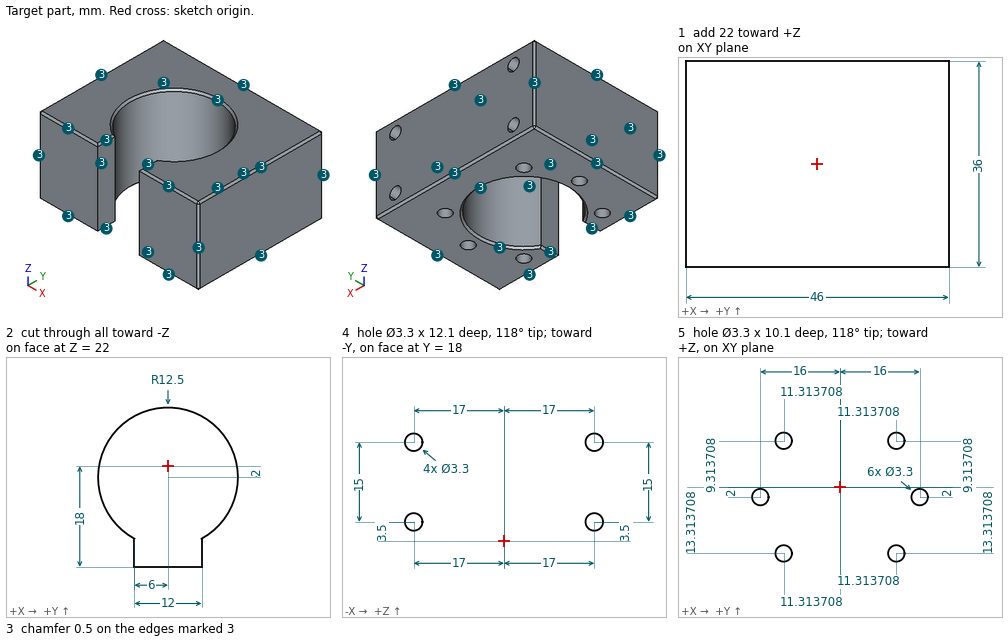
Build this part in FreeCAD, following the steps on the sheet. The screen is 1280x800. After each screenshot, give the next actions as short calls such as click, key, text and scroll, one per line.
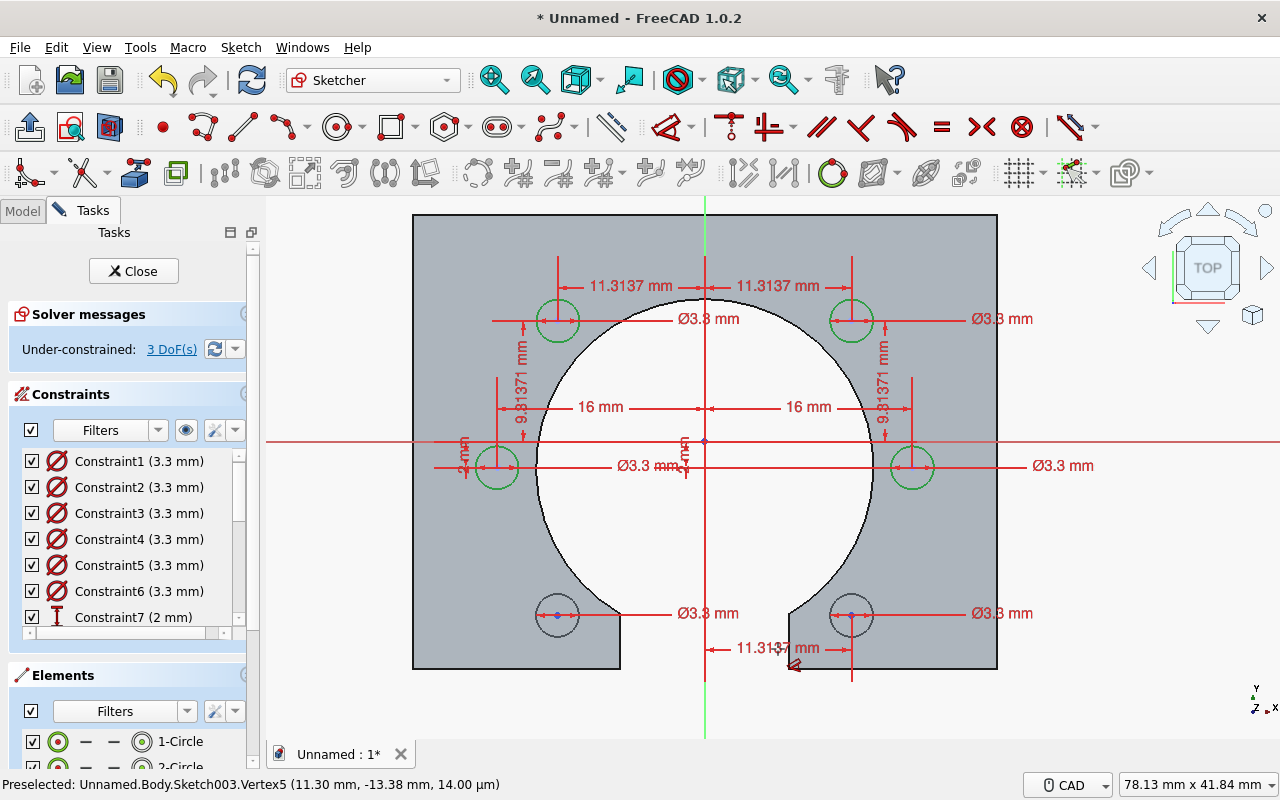
click(852, 615)
click(886, 529)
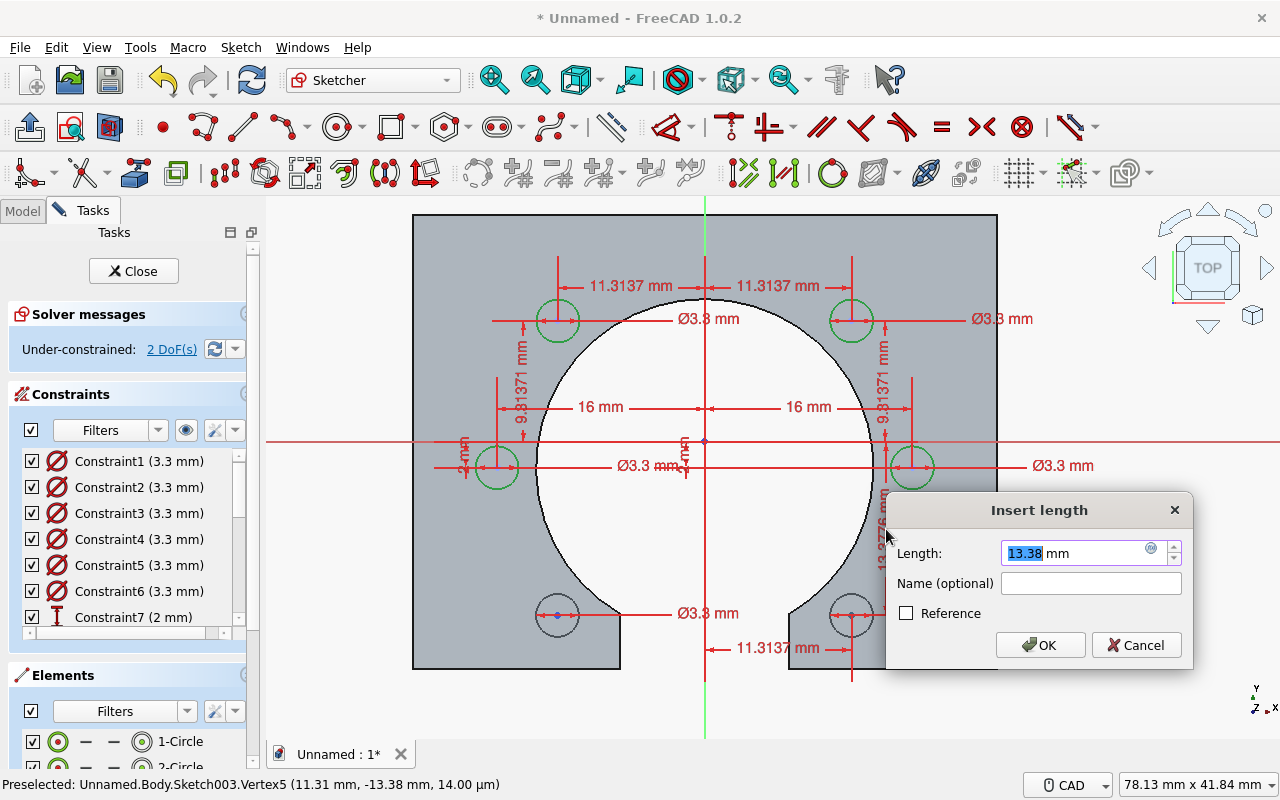
text(13.313708)
key(Return)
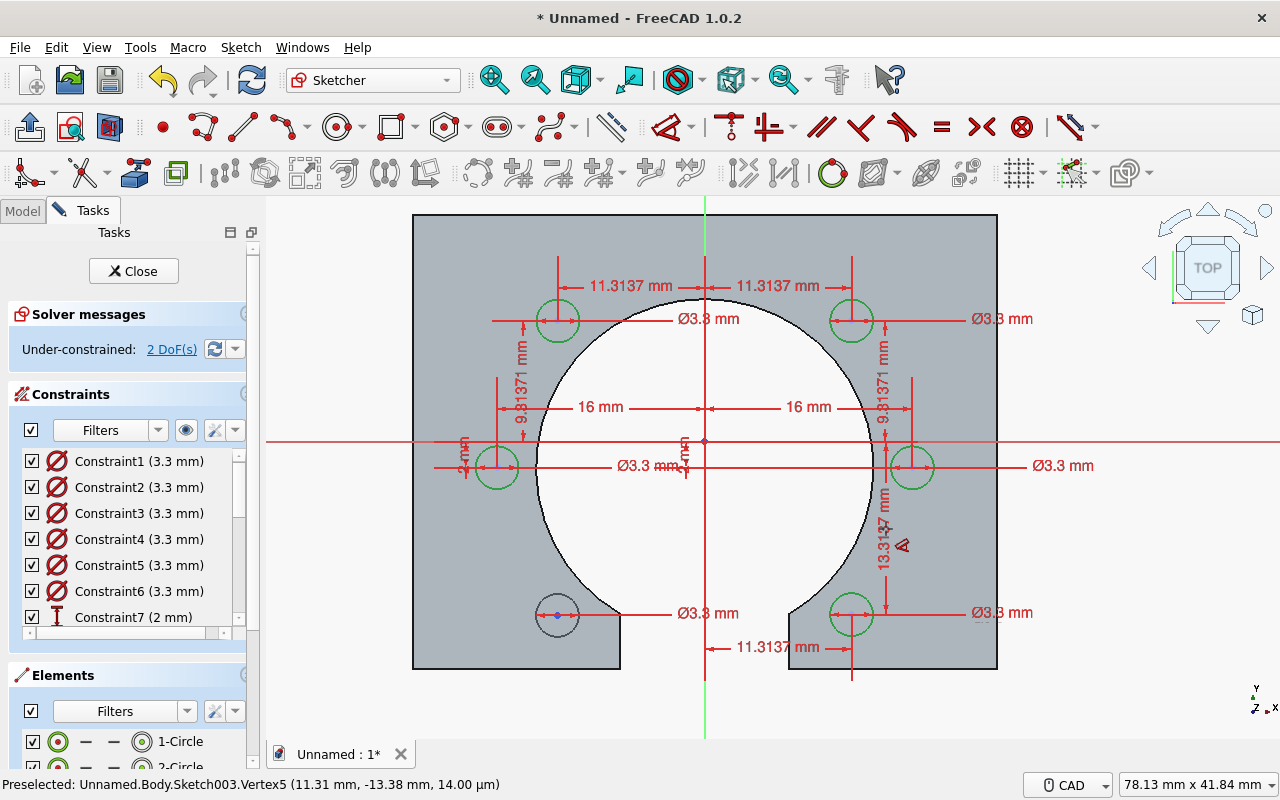
click(557, 615)
click(631, 649)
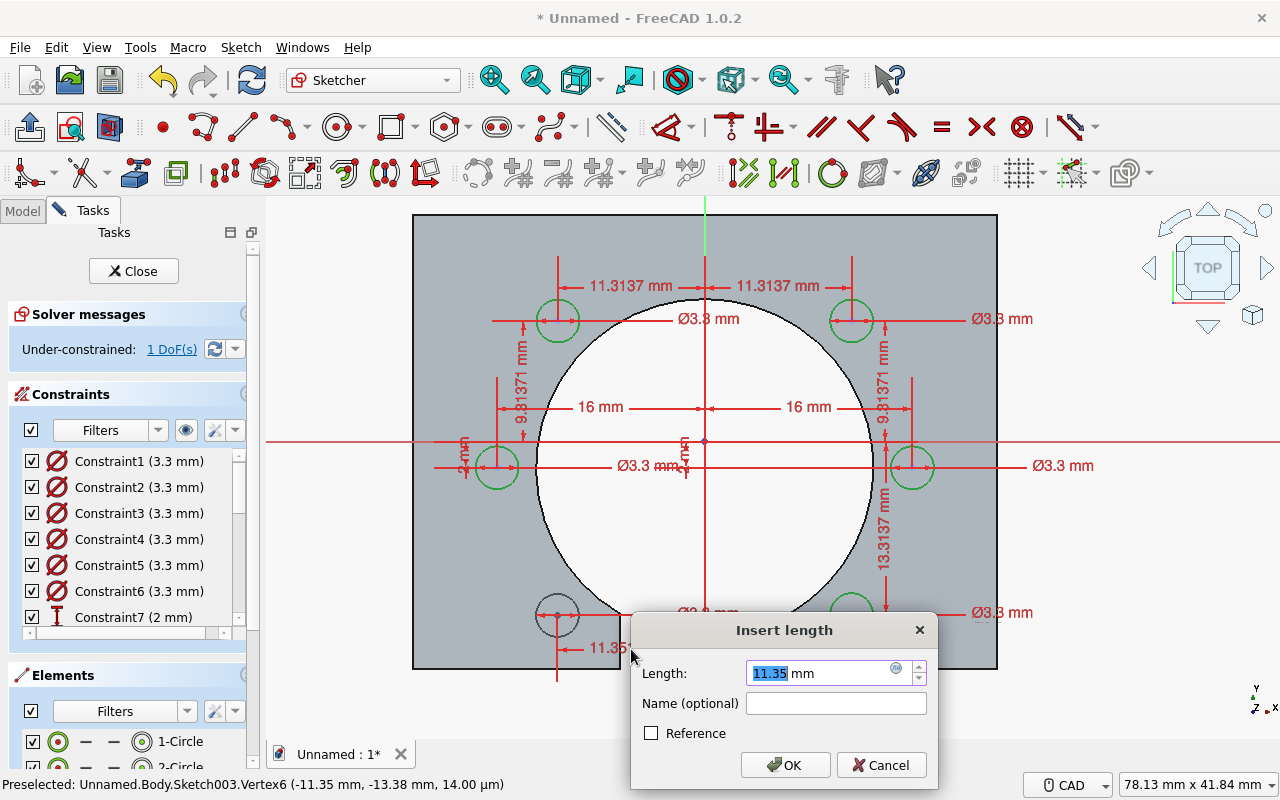
text(11.313708)
key(Return)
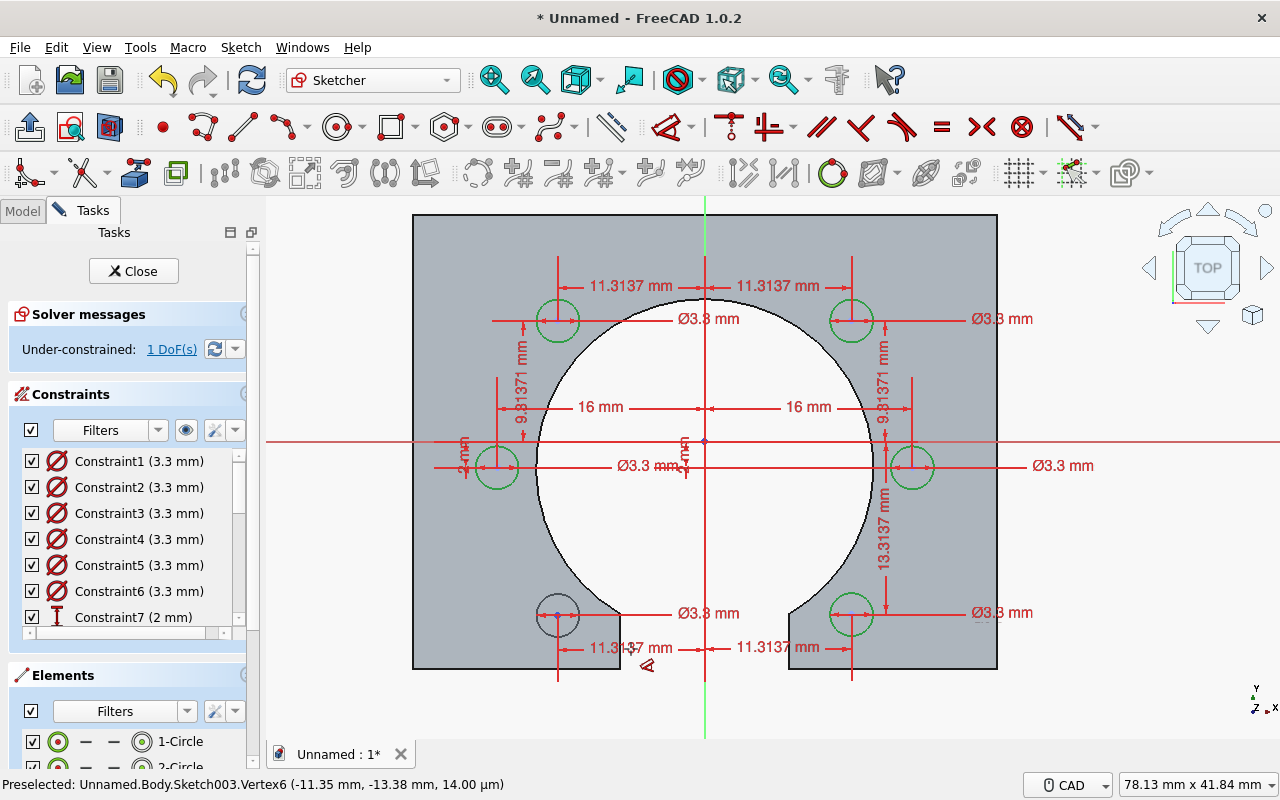
click(558, 615)
click(524, 529)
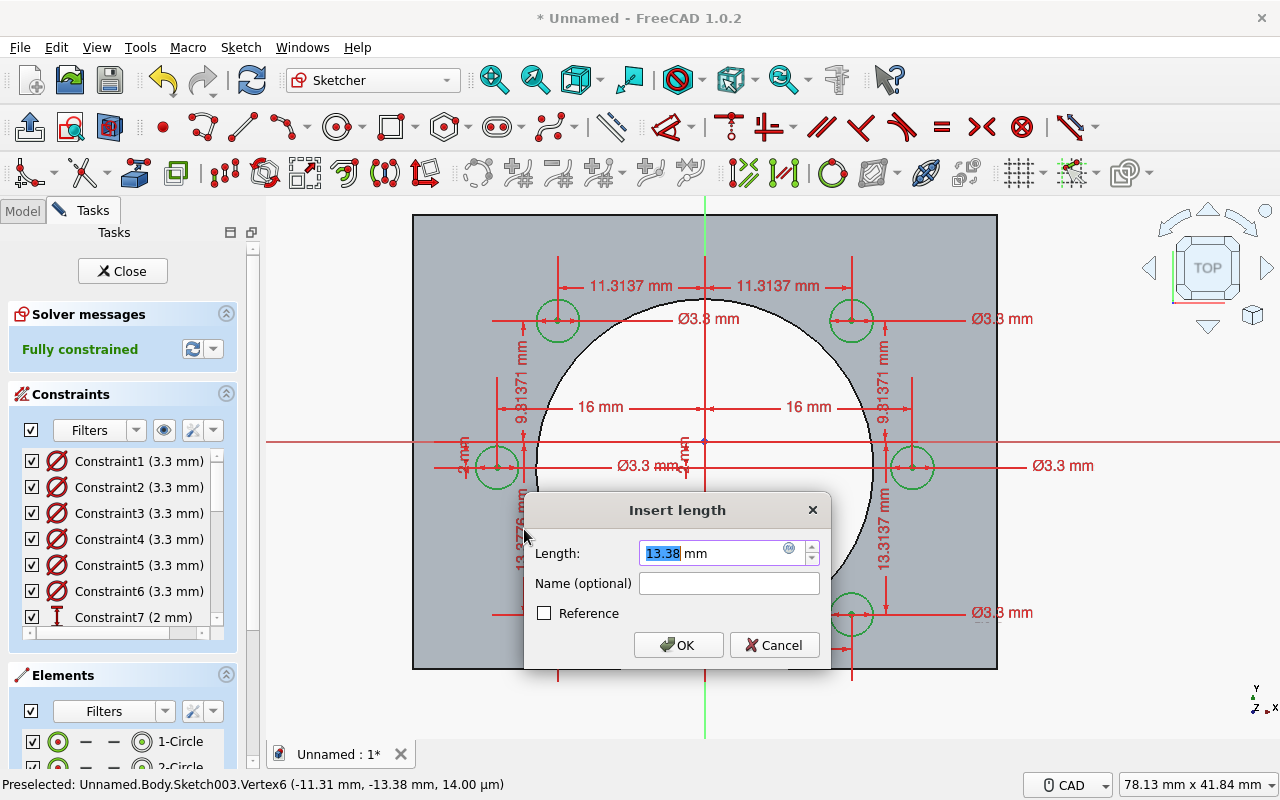
text(13.313708)
key(Return)
key(Escape)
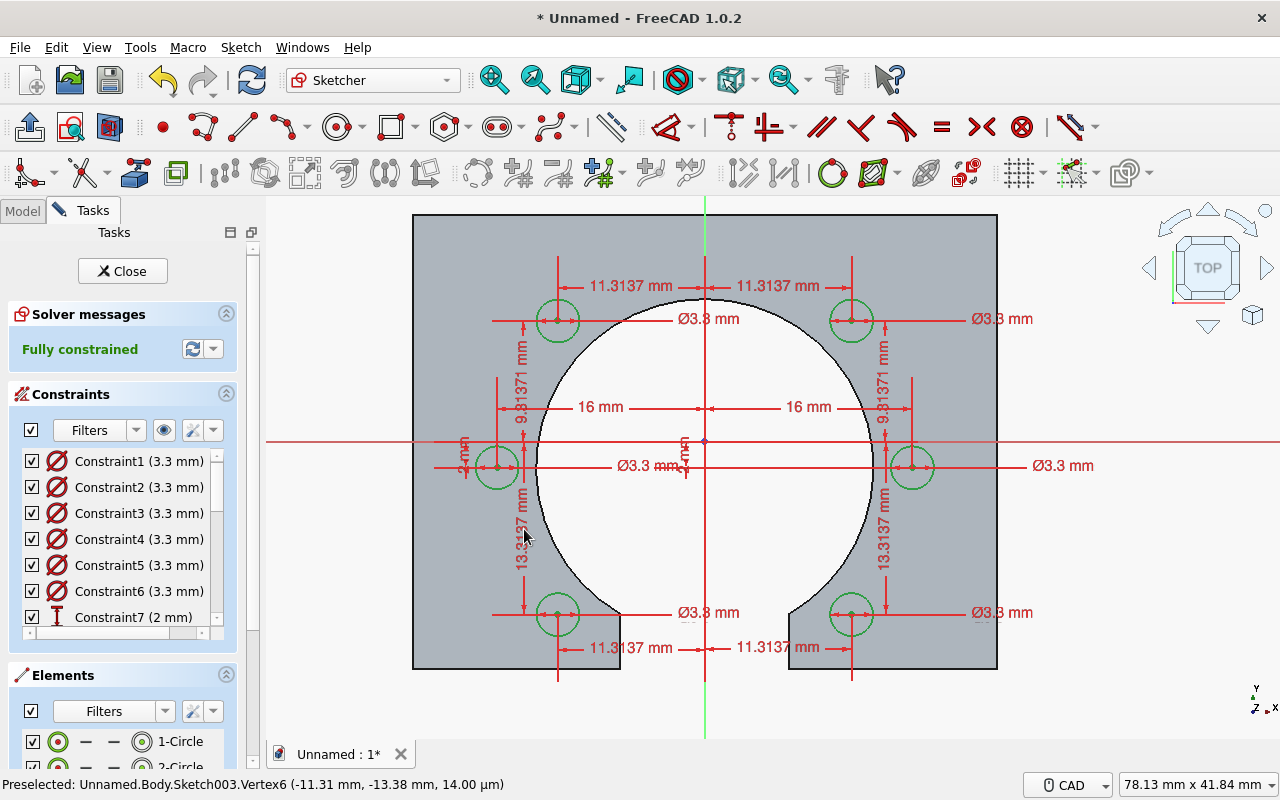
click(123, 271)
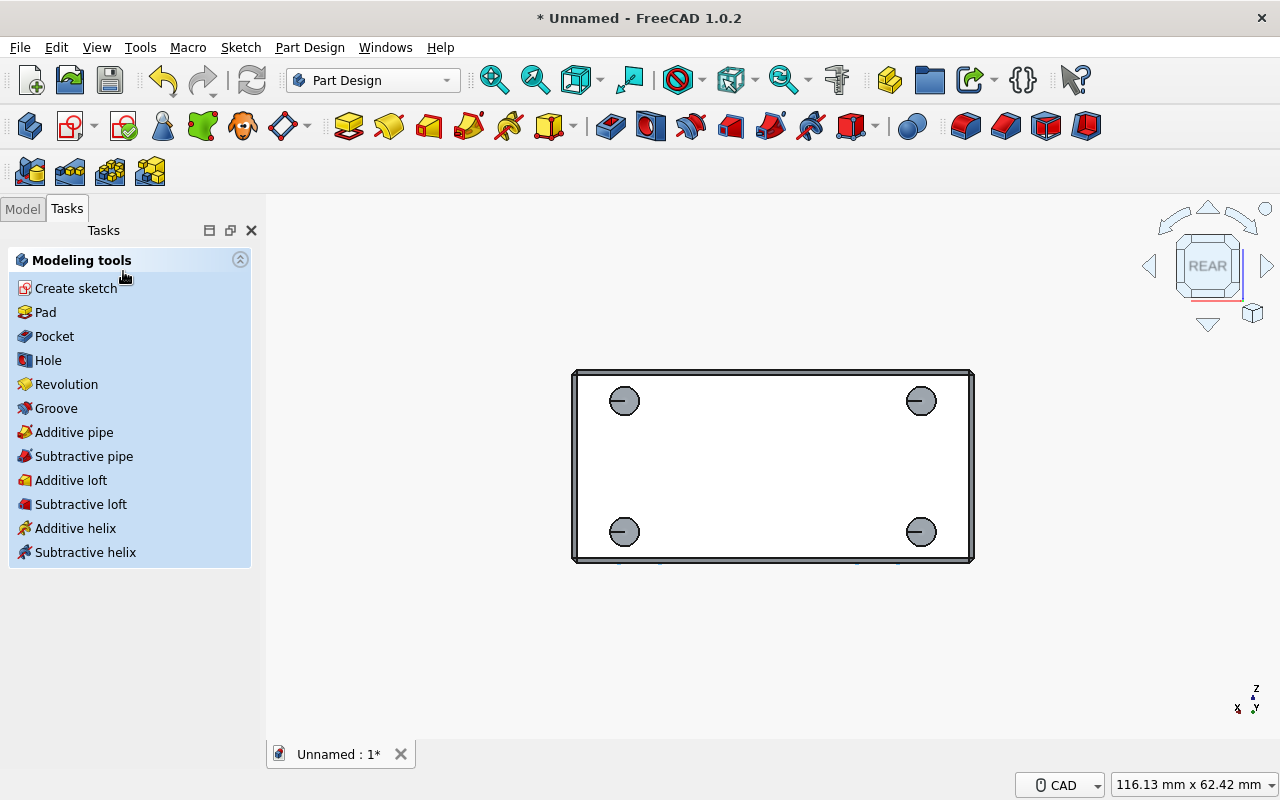
click(652, 126)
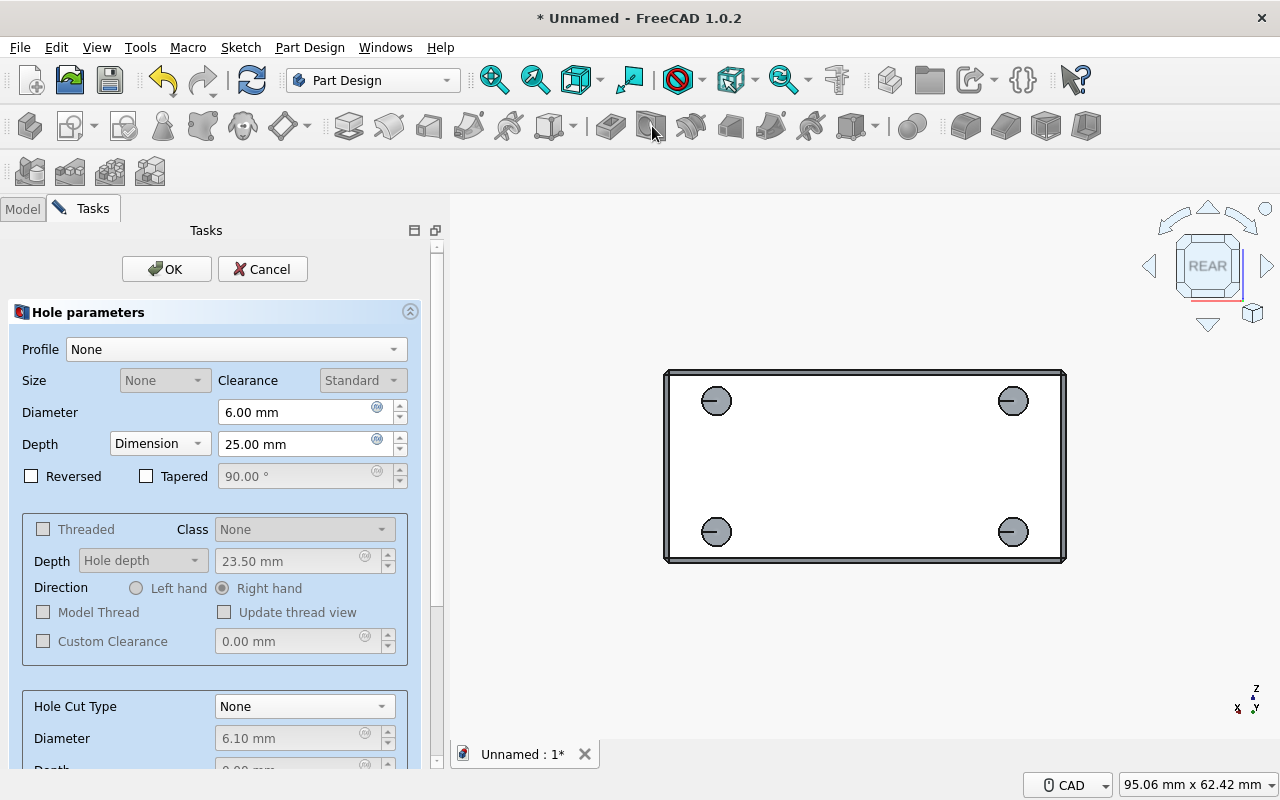
triple_click(305, 412)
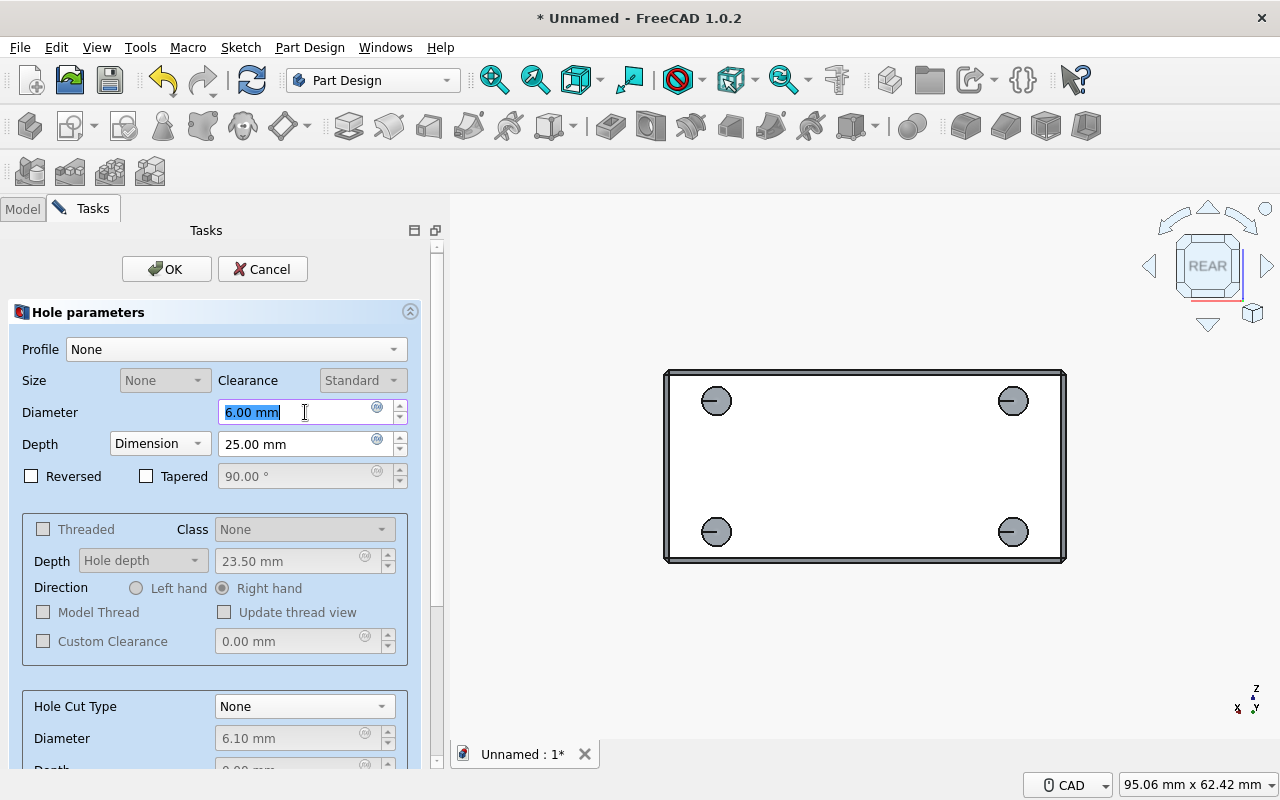
text(3.3)
key(Tab)